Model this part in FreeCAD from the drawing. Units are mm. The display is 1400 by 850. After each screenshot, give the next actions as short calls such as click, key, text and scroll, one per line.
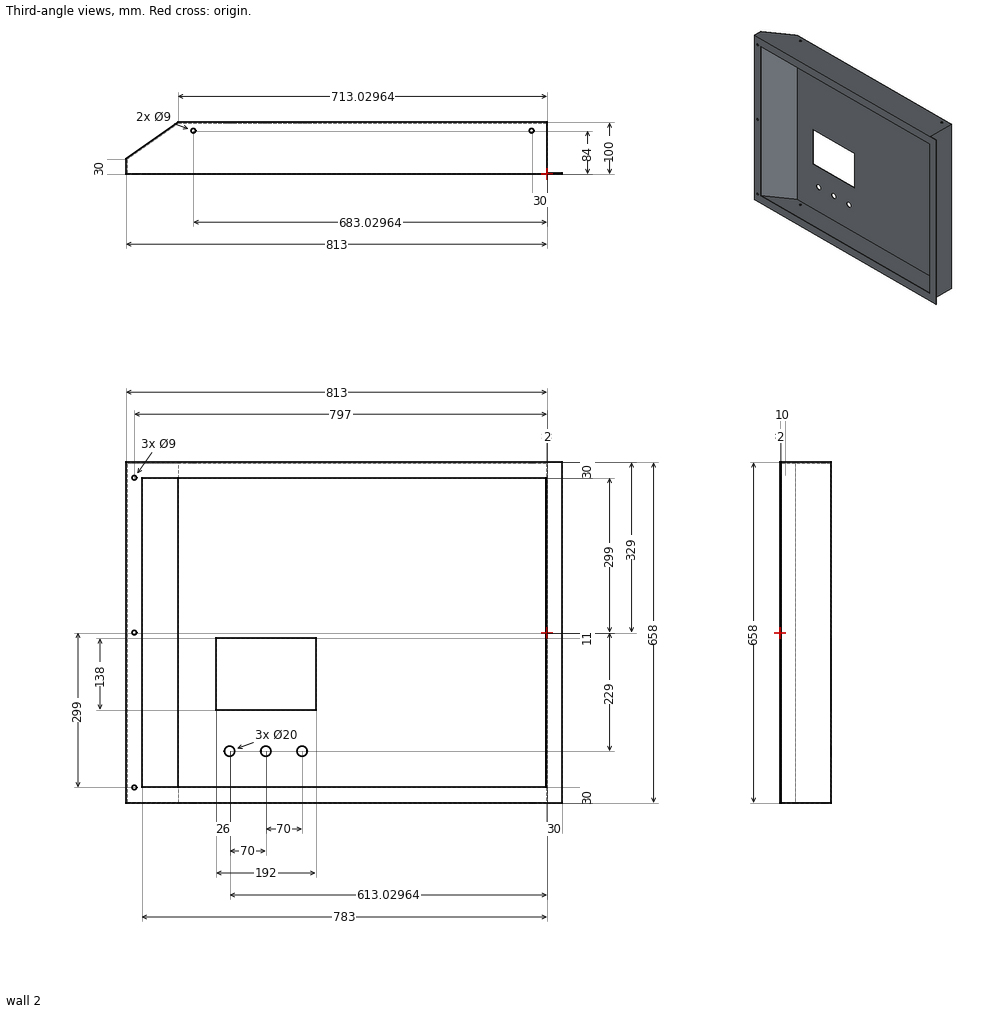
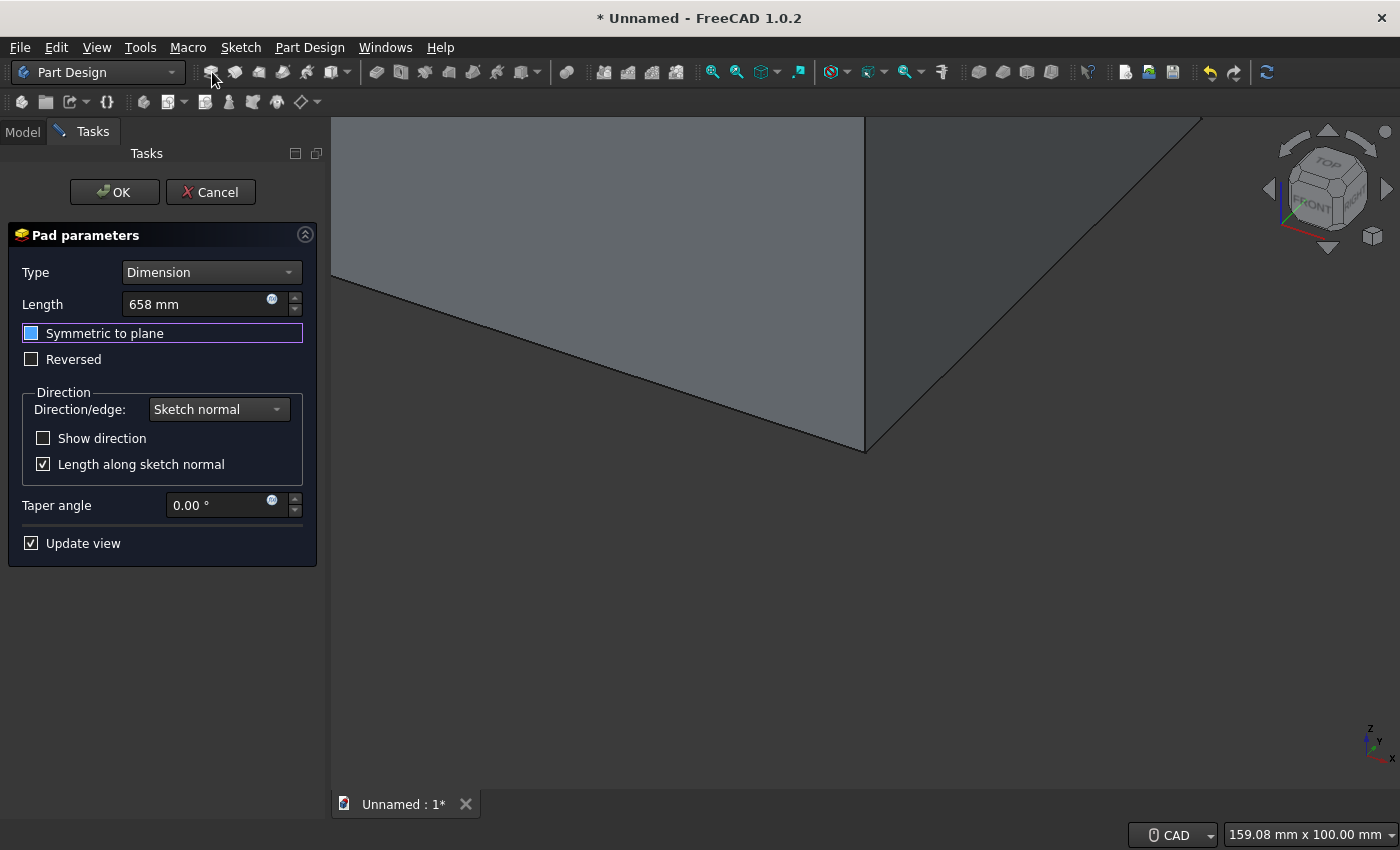
click(30, 333)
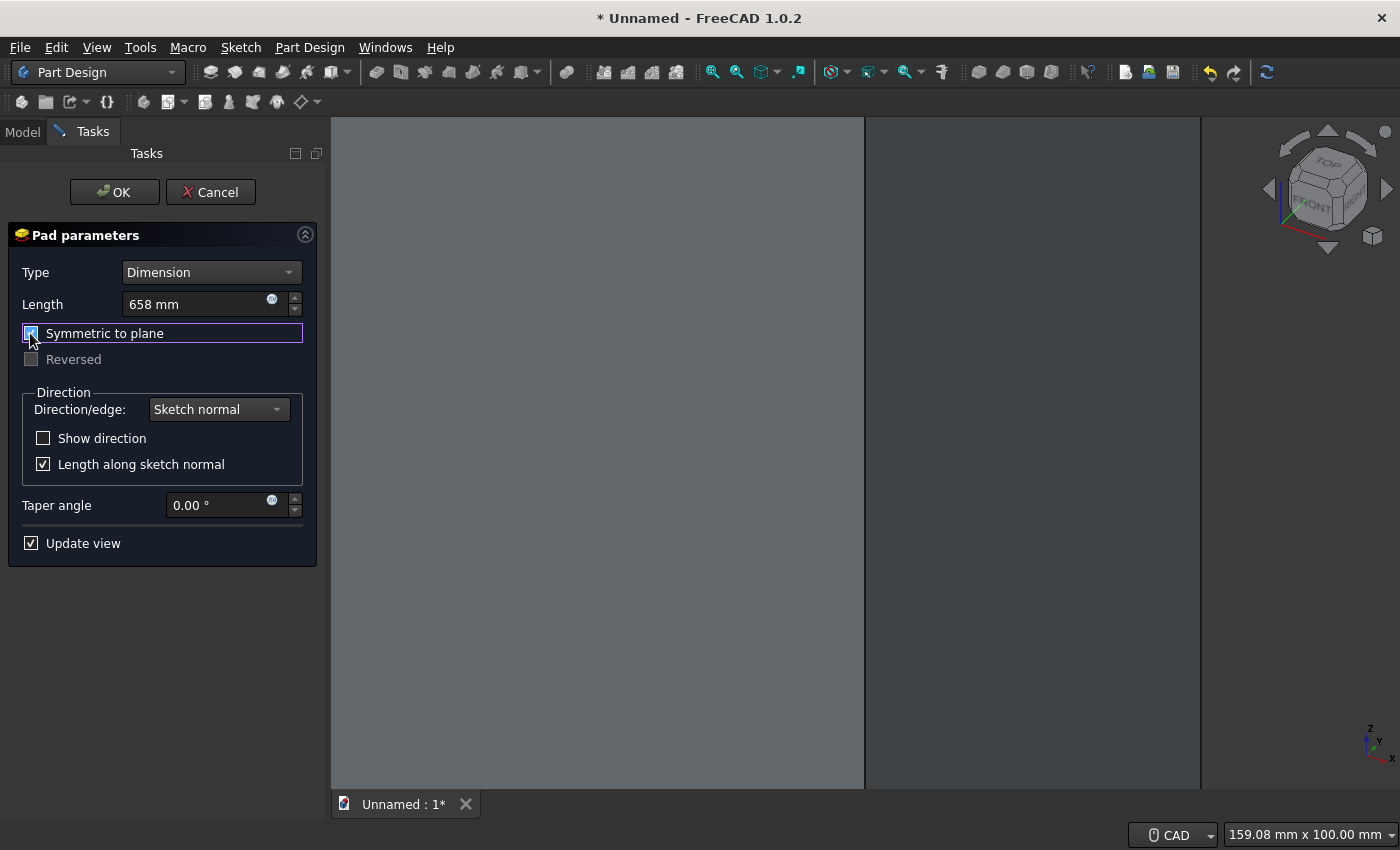
click(115, 192)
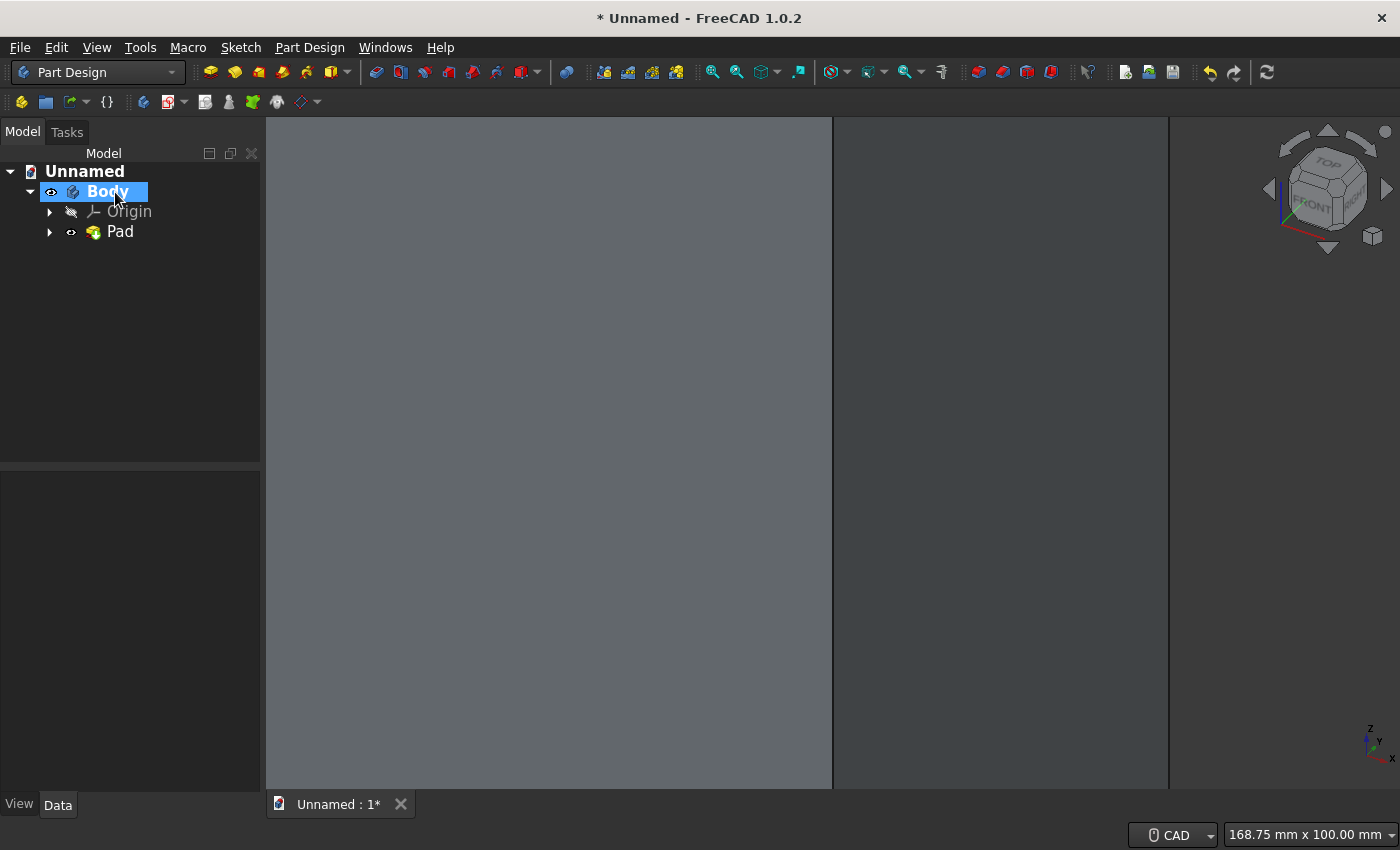
key(v)
key(f)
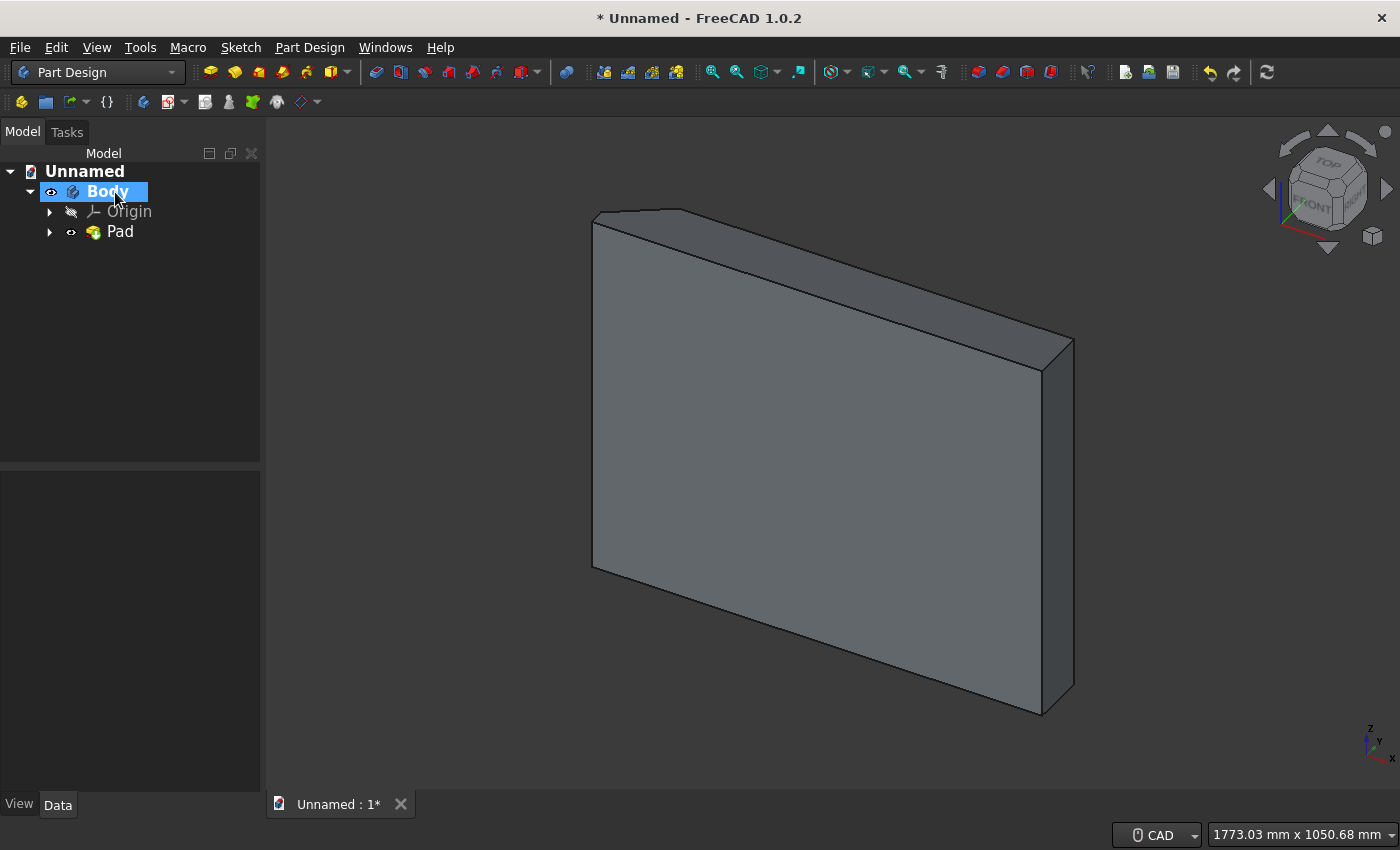
click(817, 468)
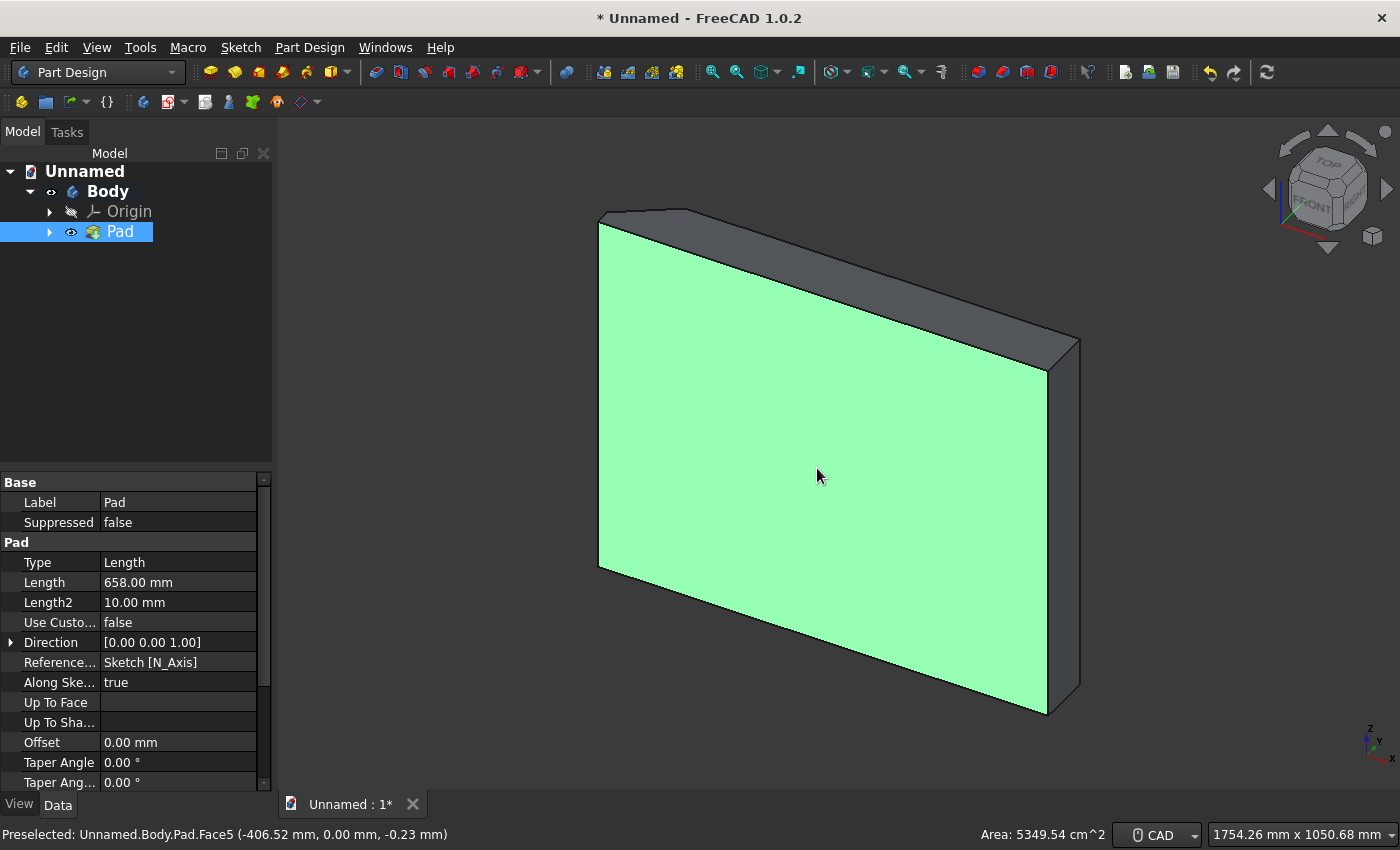
click(1052, 72)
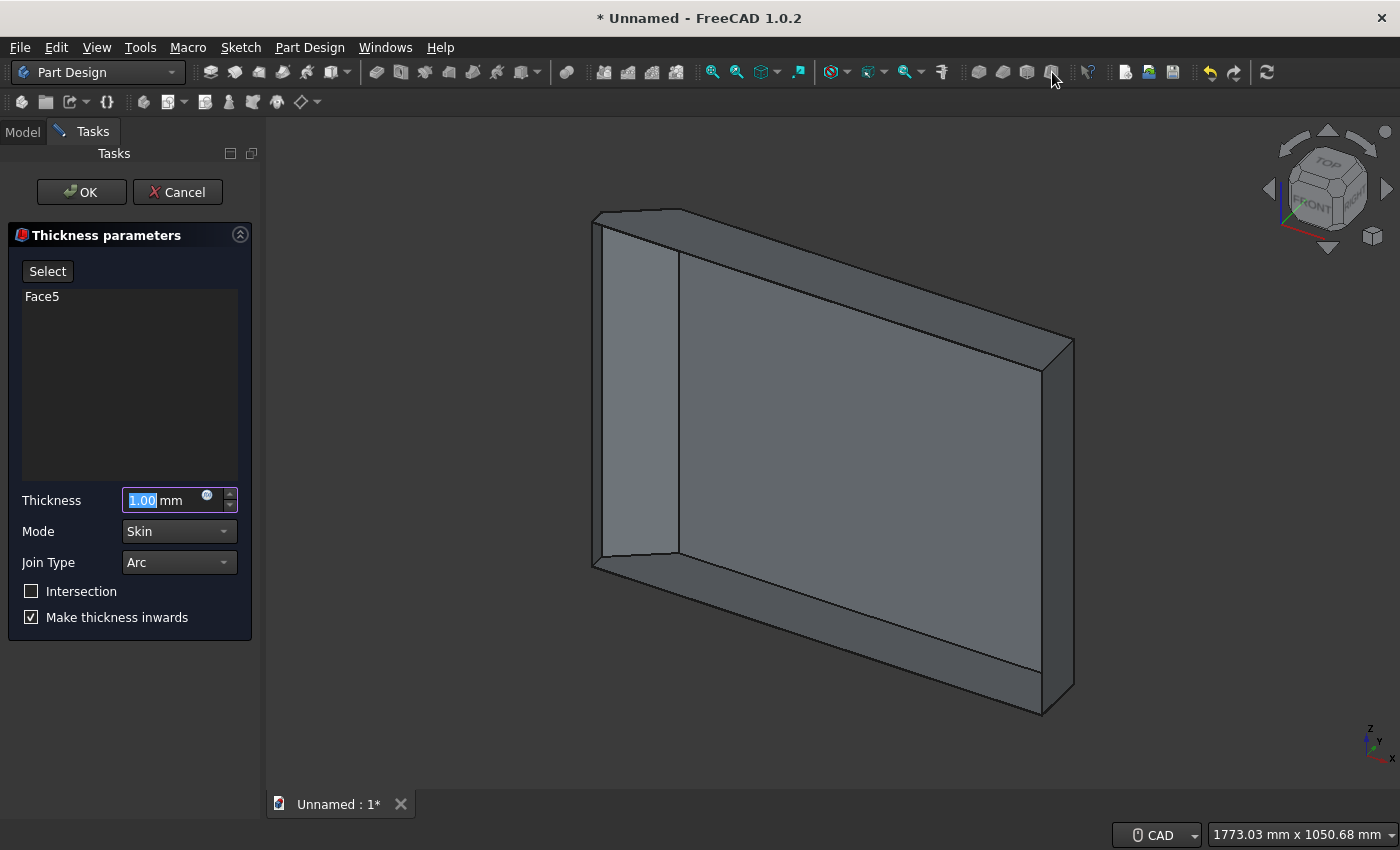
text(2)
key(Tab)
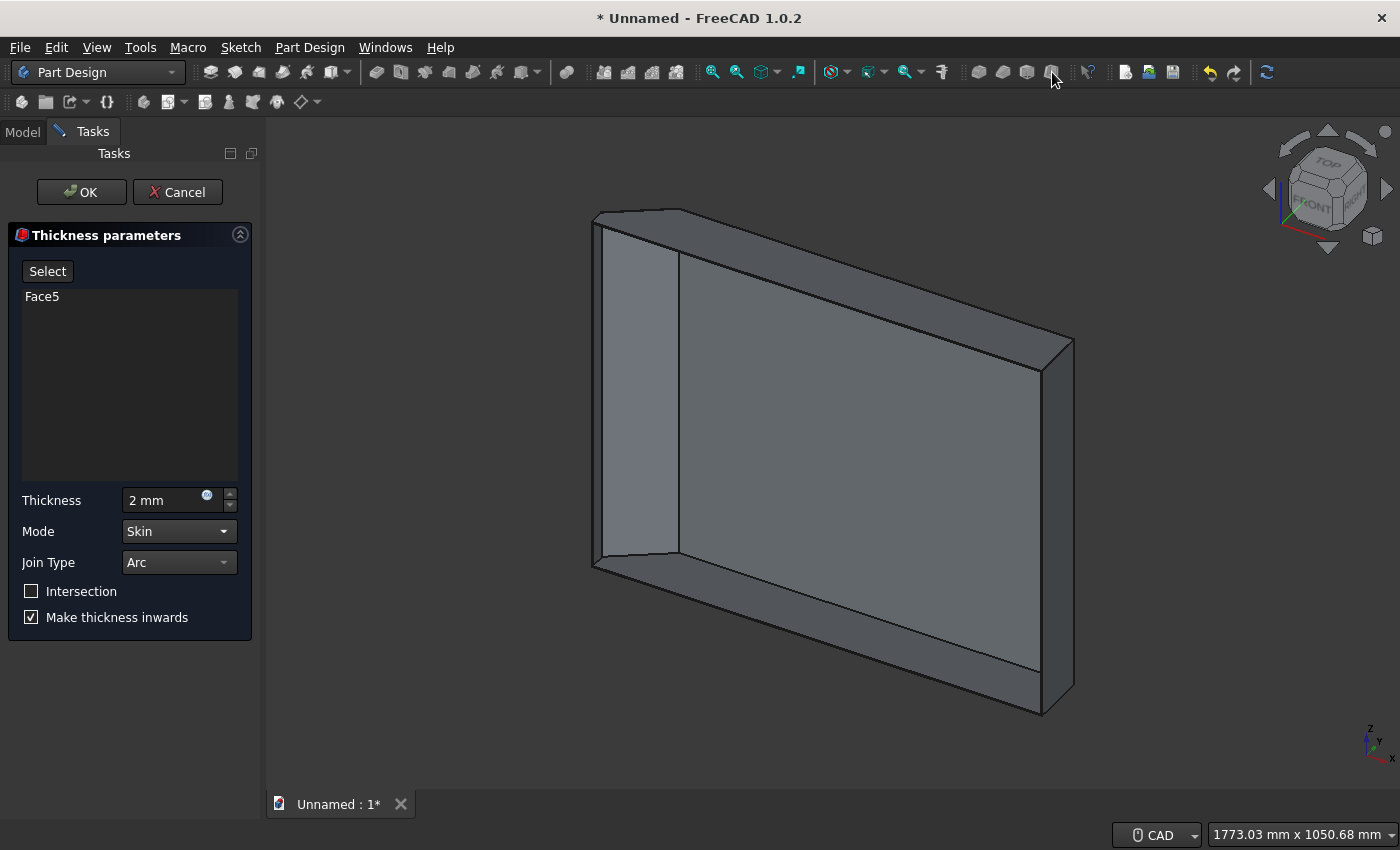
click(180, 562)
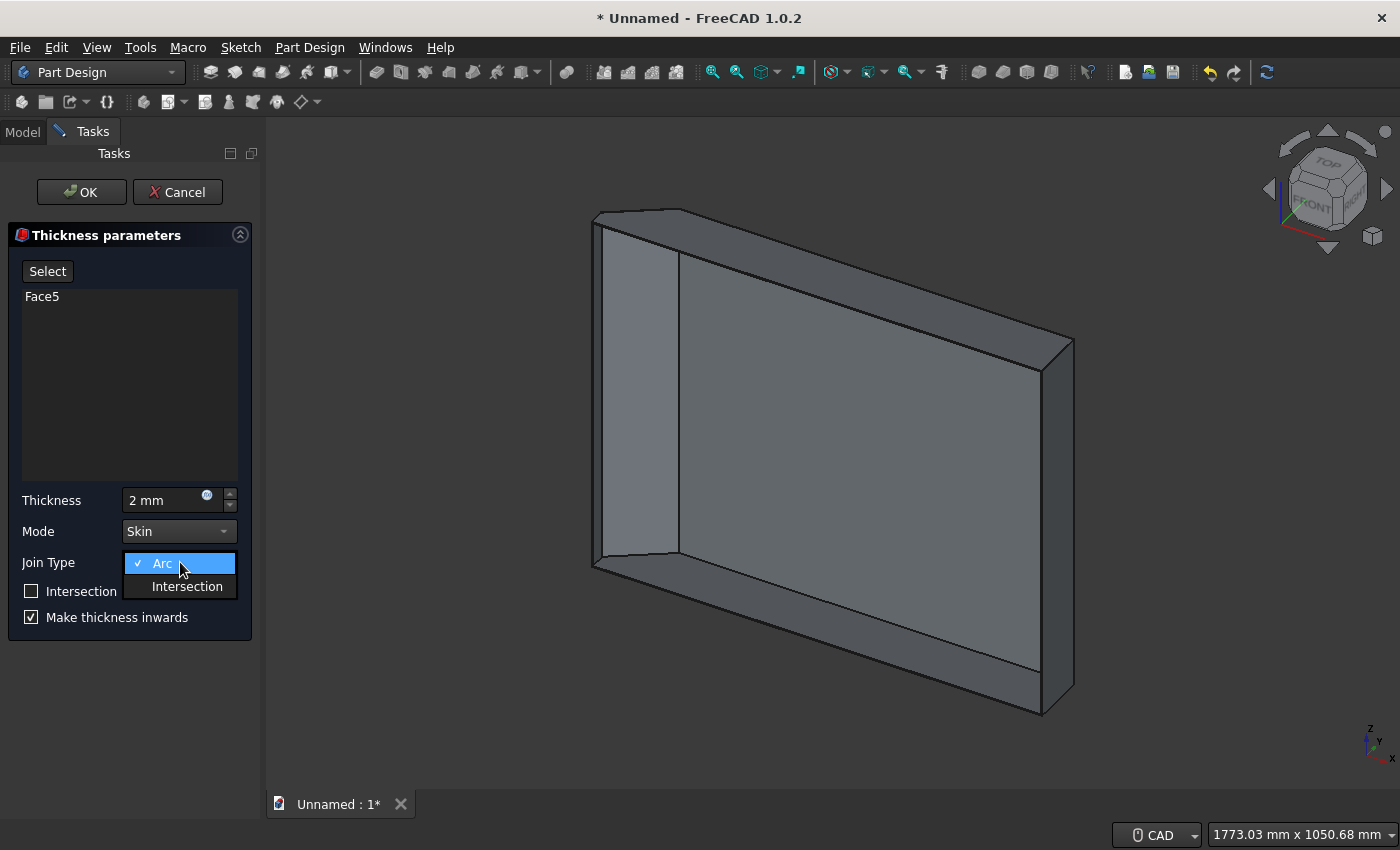
click(179, 586)